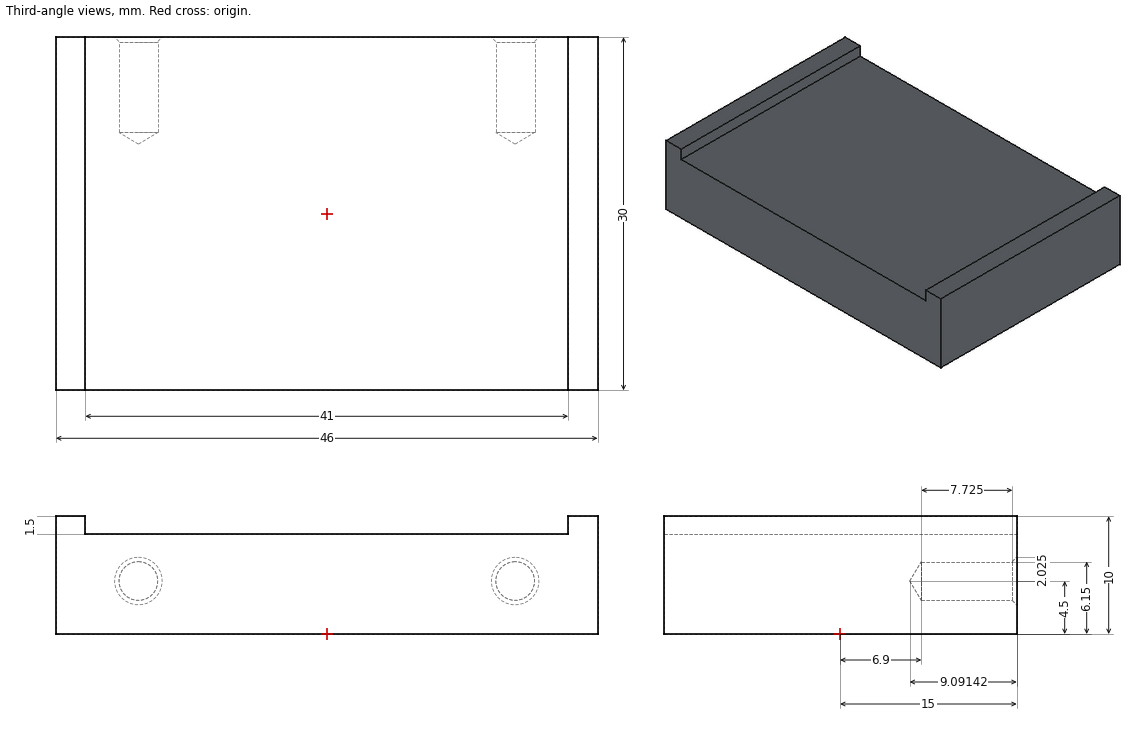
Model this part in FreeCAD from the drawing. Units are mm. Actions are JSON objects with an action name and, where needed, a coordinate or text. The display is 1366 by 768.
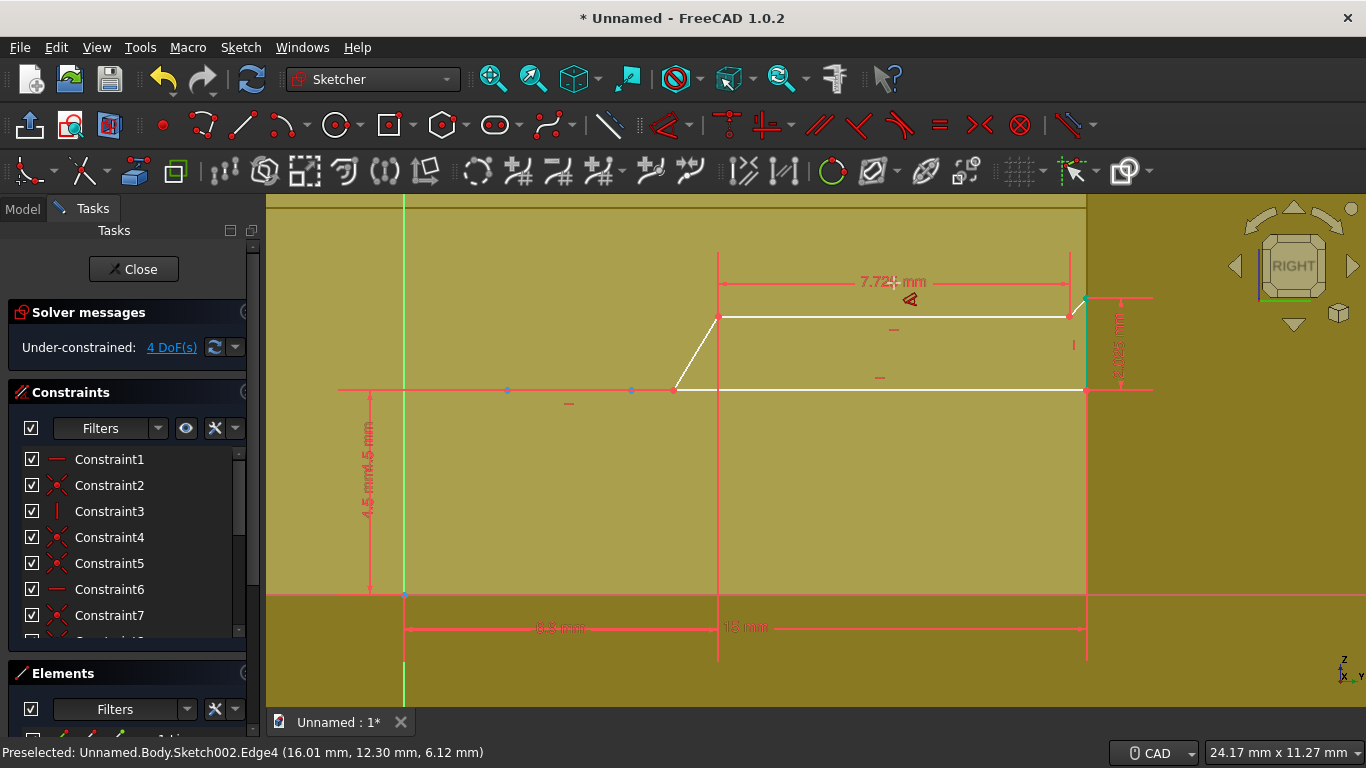
{"action": "left_click", "coordinate": [1070, 317]}
{"action": "left_click", "coordinate": [370, 392]}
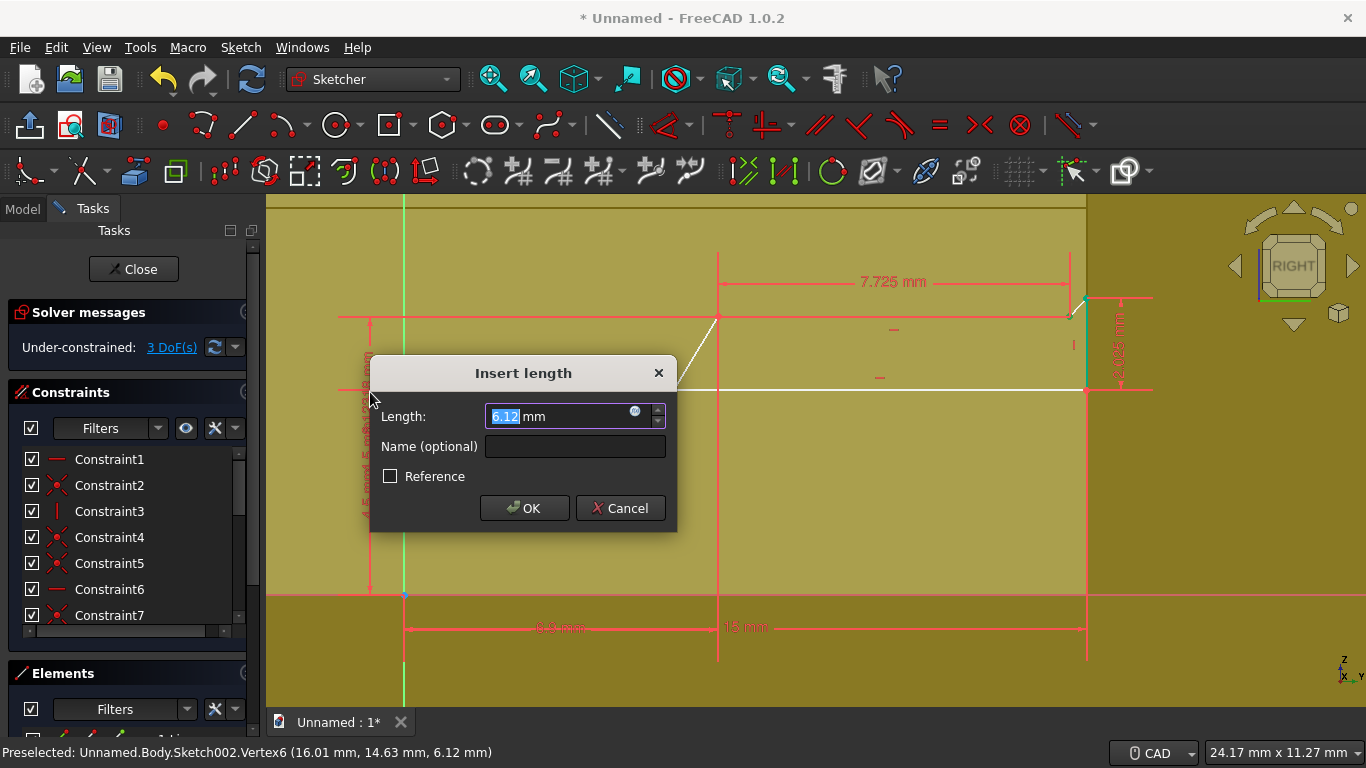
{"action": "type", "text": "6.15"}
{"action": "key", "text": "Return"}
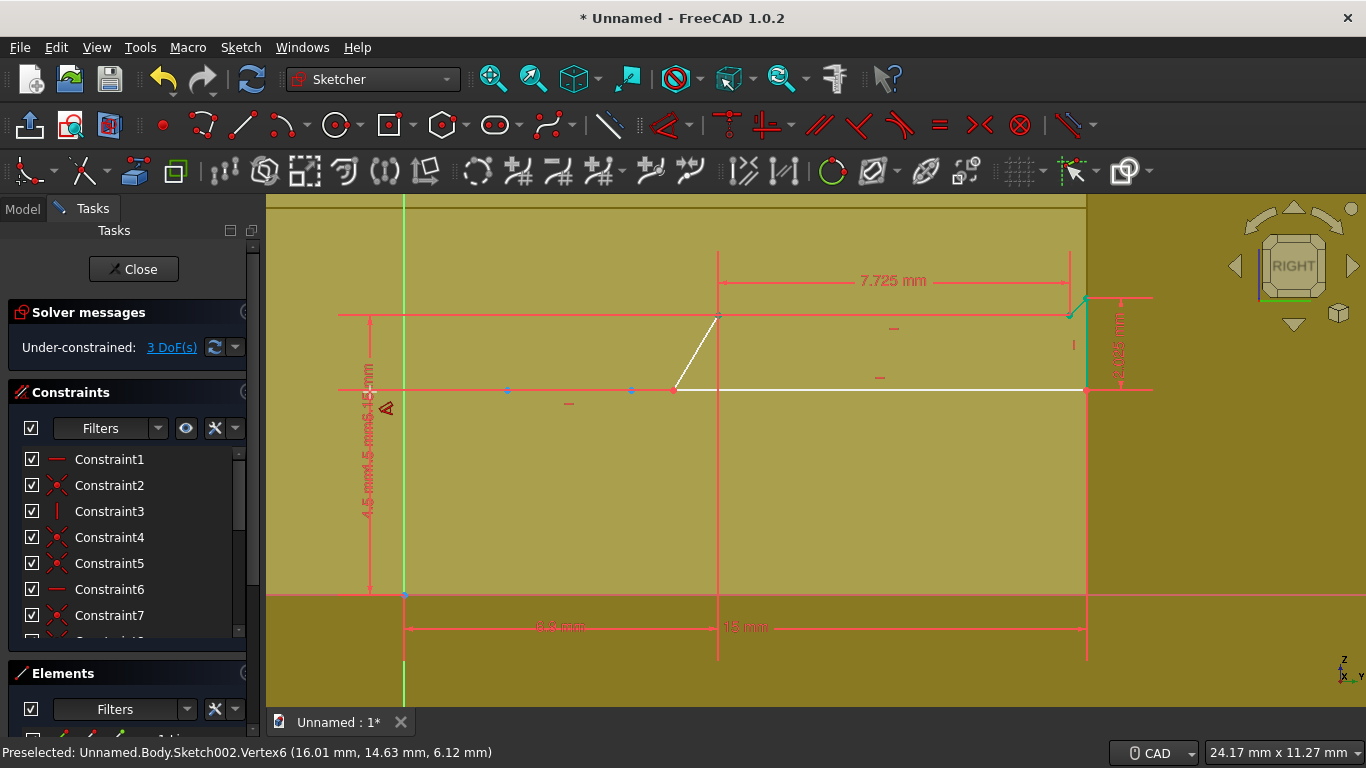
{"action": "left_click", "coordinate": [798, 390]}
{"action": "left_click", "coordinate": [880, 356]}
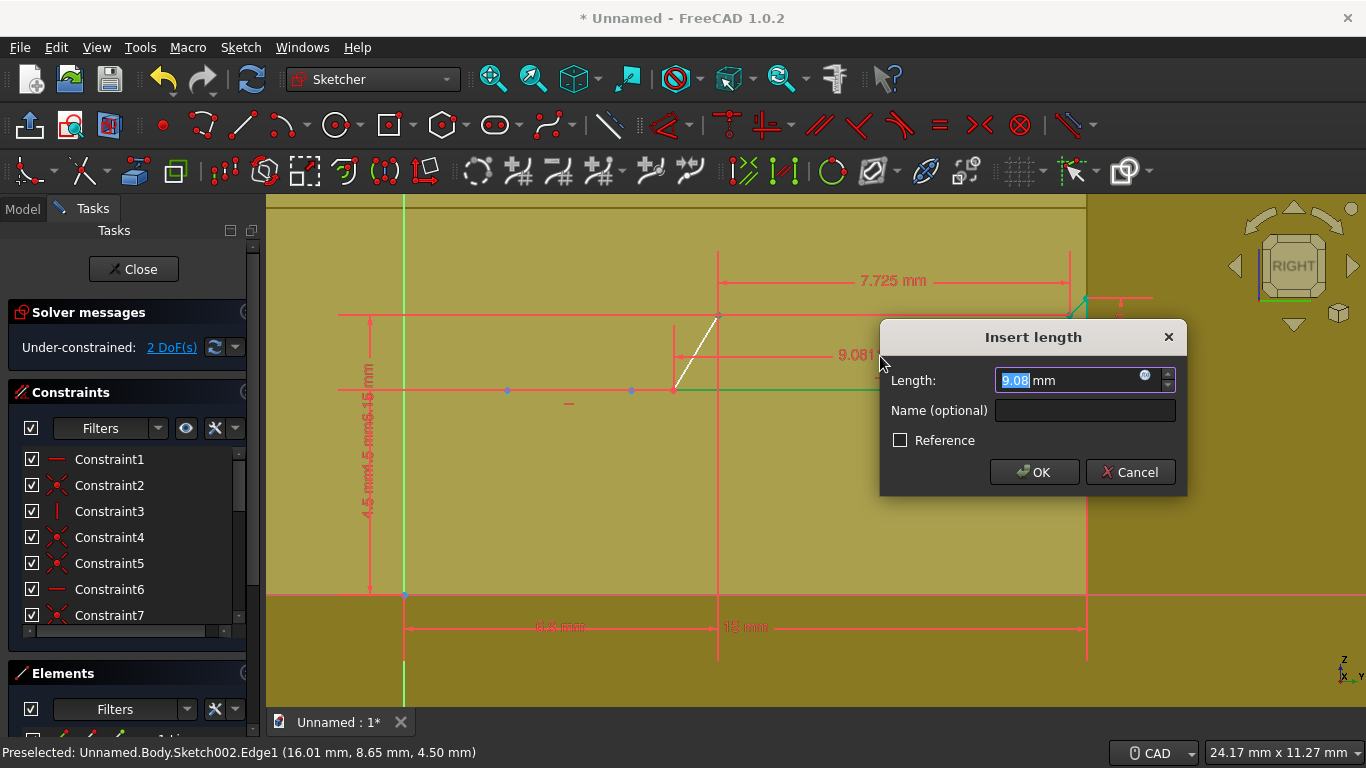
{"action": "type", "text": "9.09142"}
{"action": "key", "text": "Return"}
{"action": "key", "text": "Escape"}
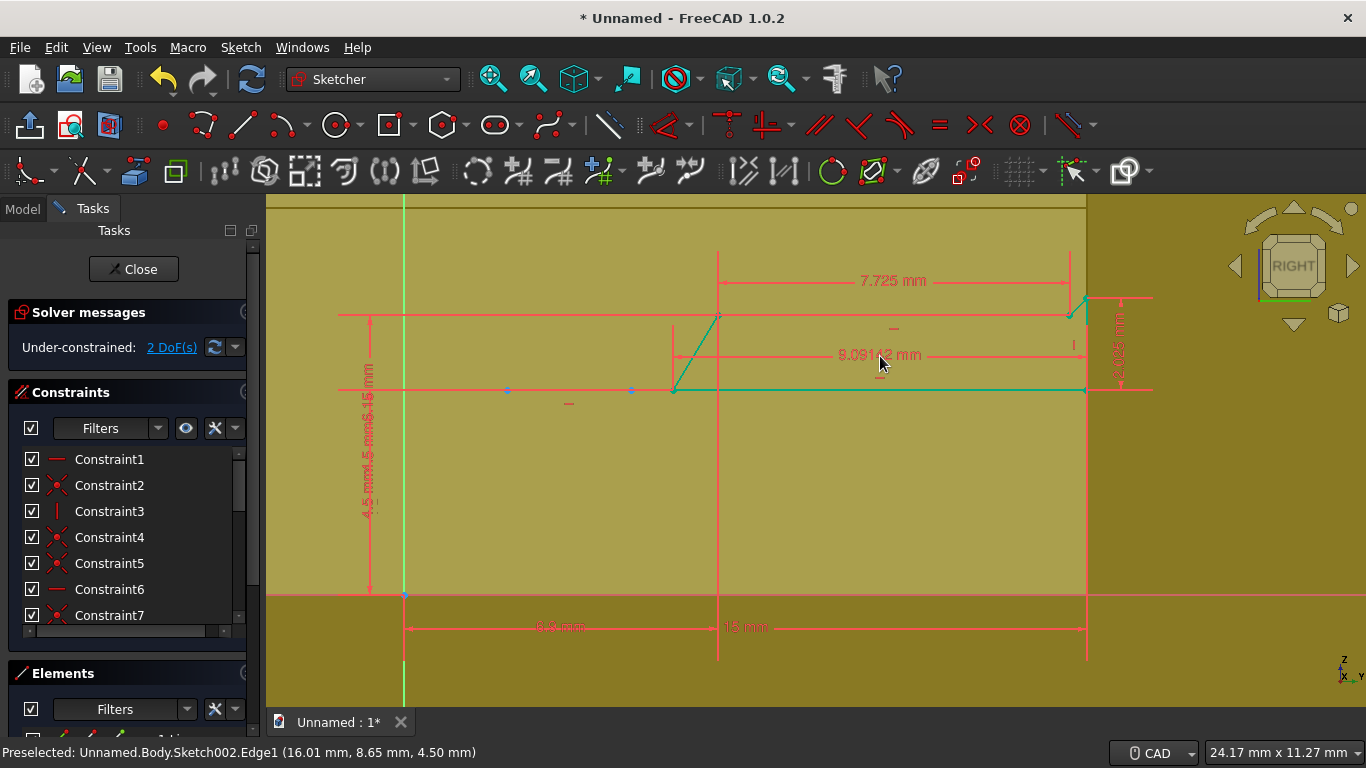
{"action": "left_click", "coordinate": [134, 269]}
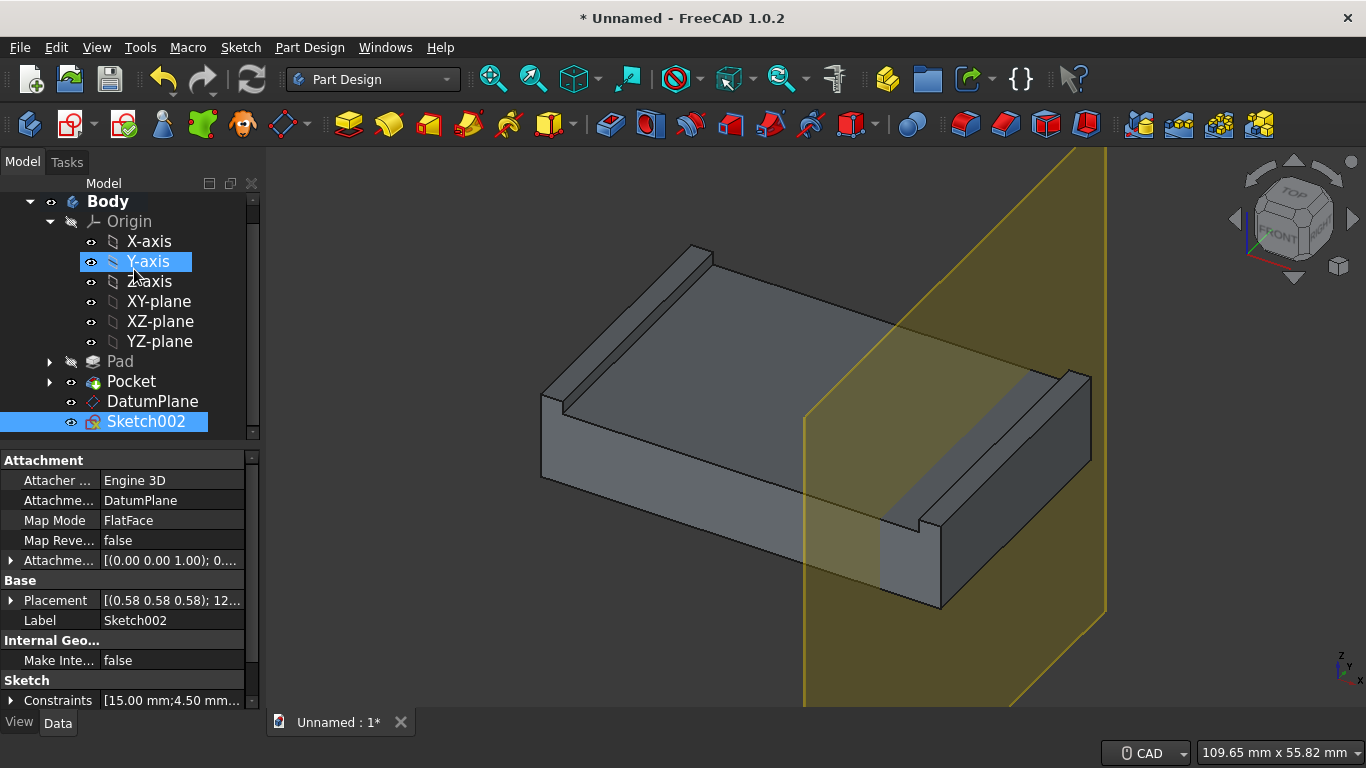
{"action": "left_click", "coordinate": [692, 124]}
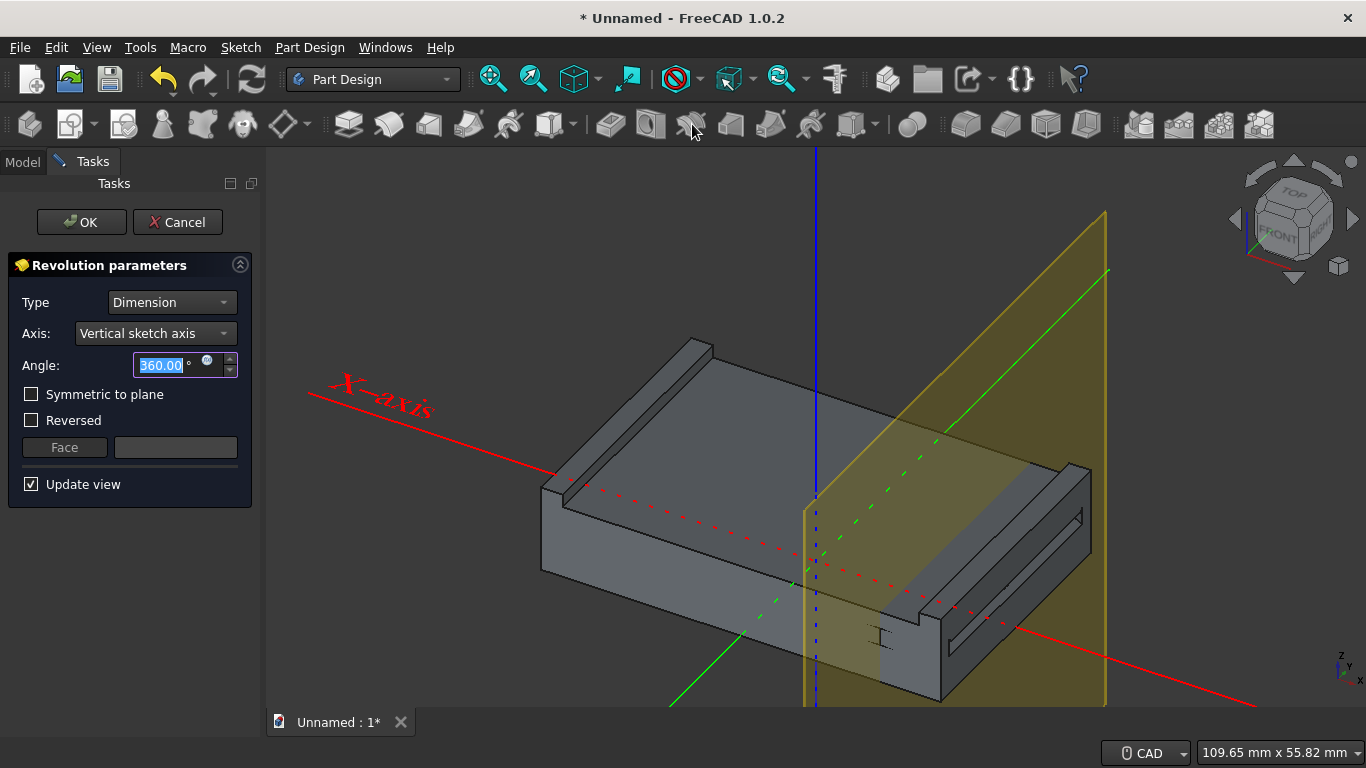
{"action": "left_click", "coordinate": [156, 334]}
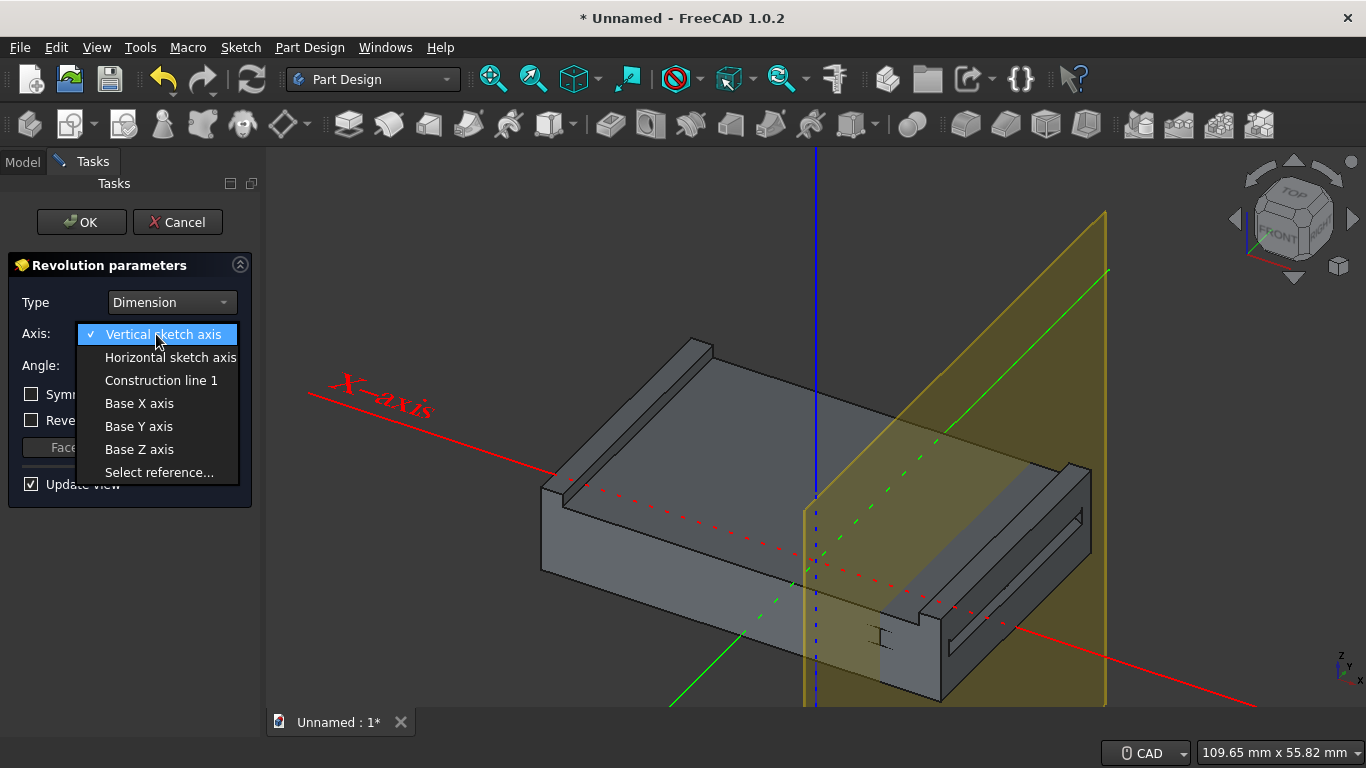
{"action": "left_click", "coordinate": [156, 380]}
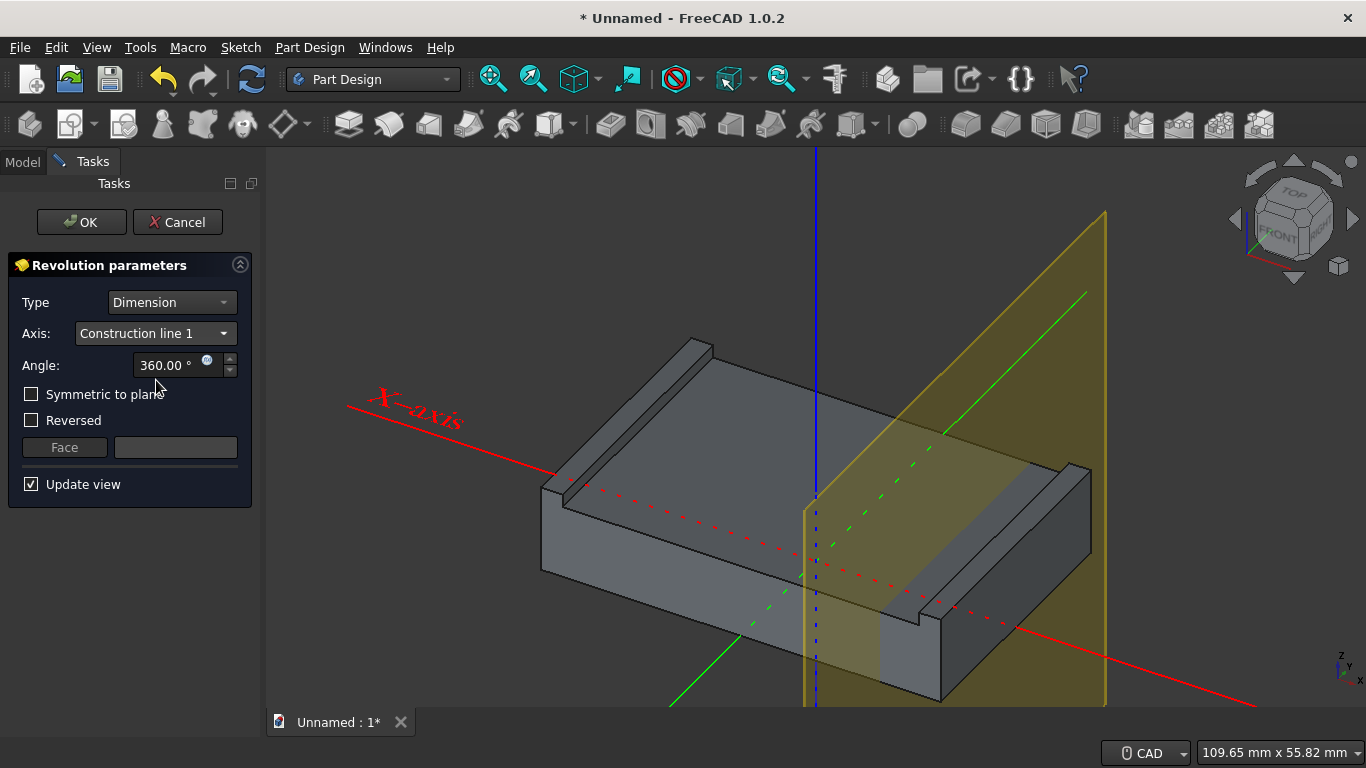
{"action": "left_click", "coordinate": [82, 222]}